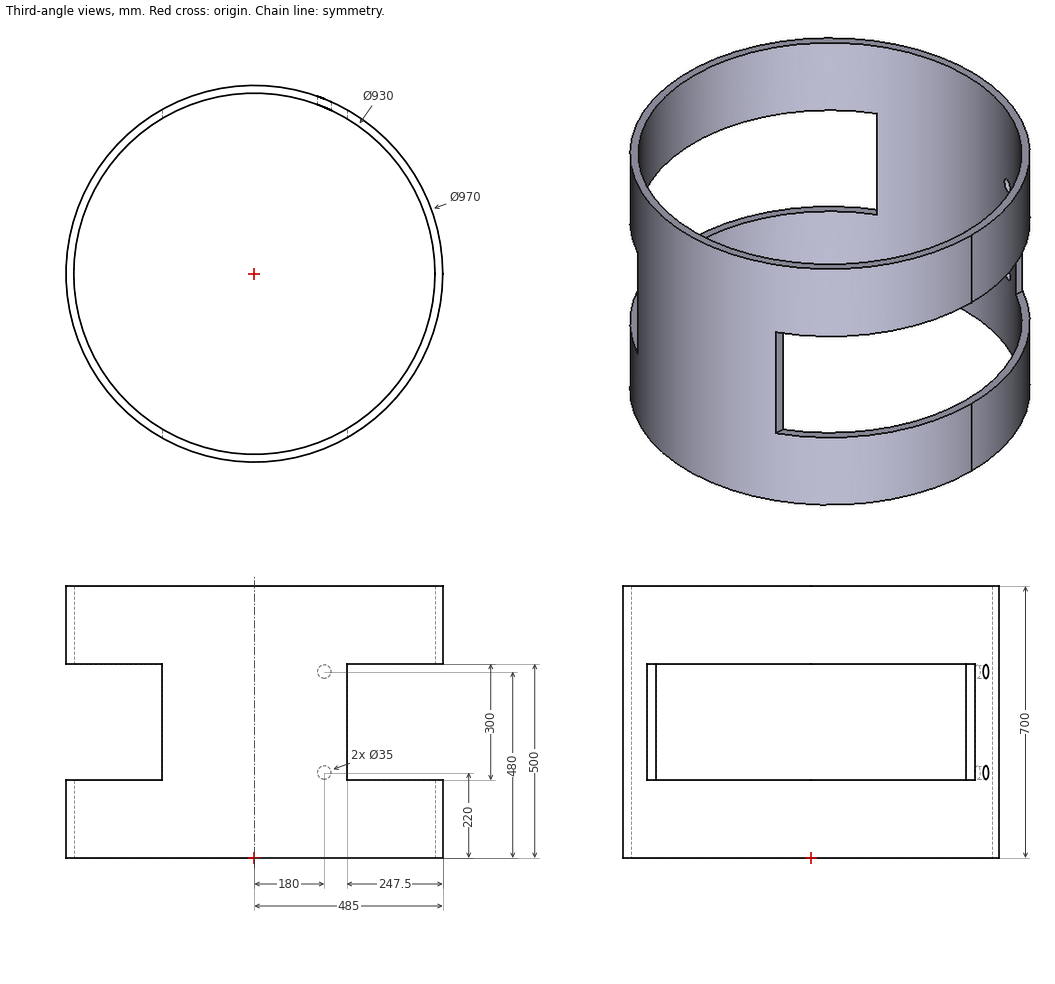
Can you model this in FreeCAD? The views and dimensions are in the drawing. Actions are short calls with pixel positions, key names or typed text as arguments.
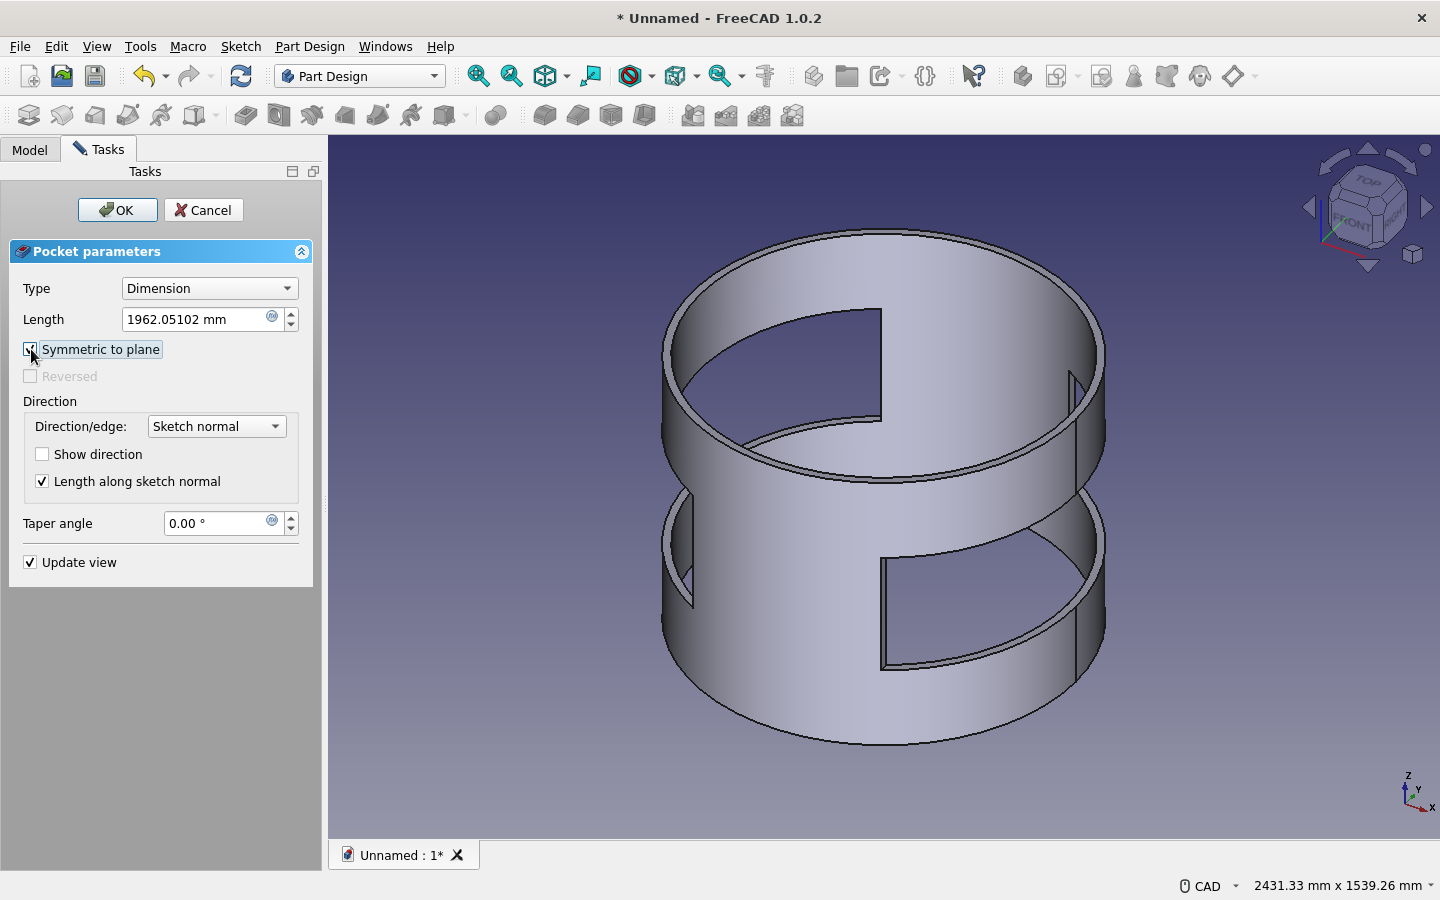
click(118, 210)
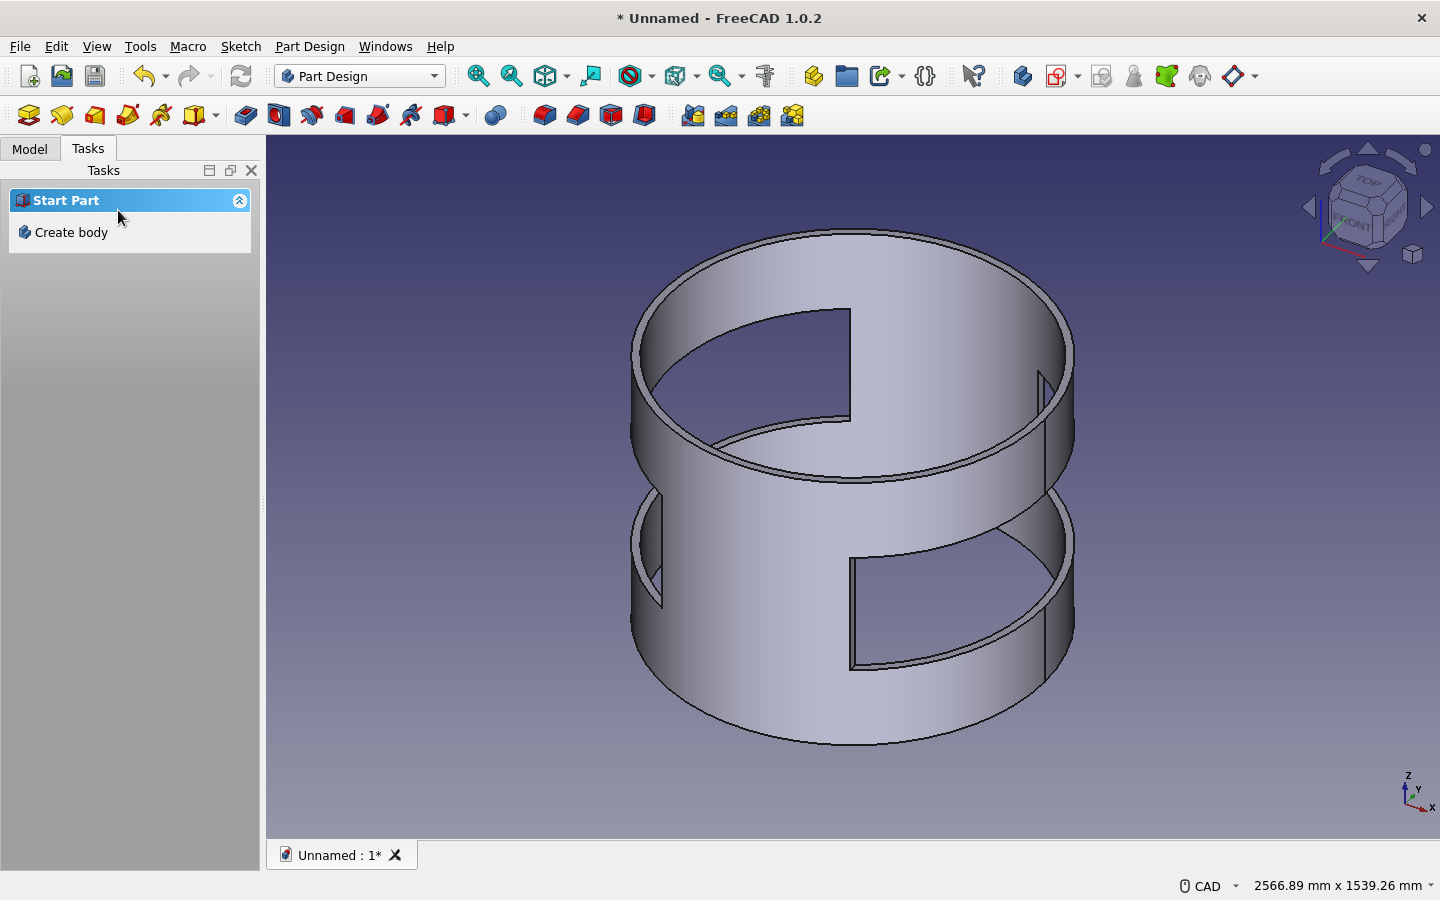
click(1056, 76)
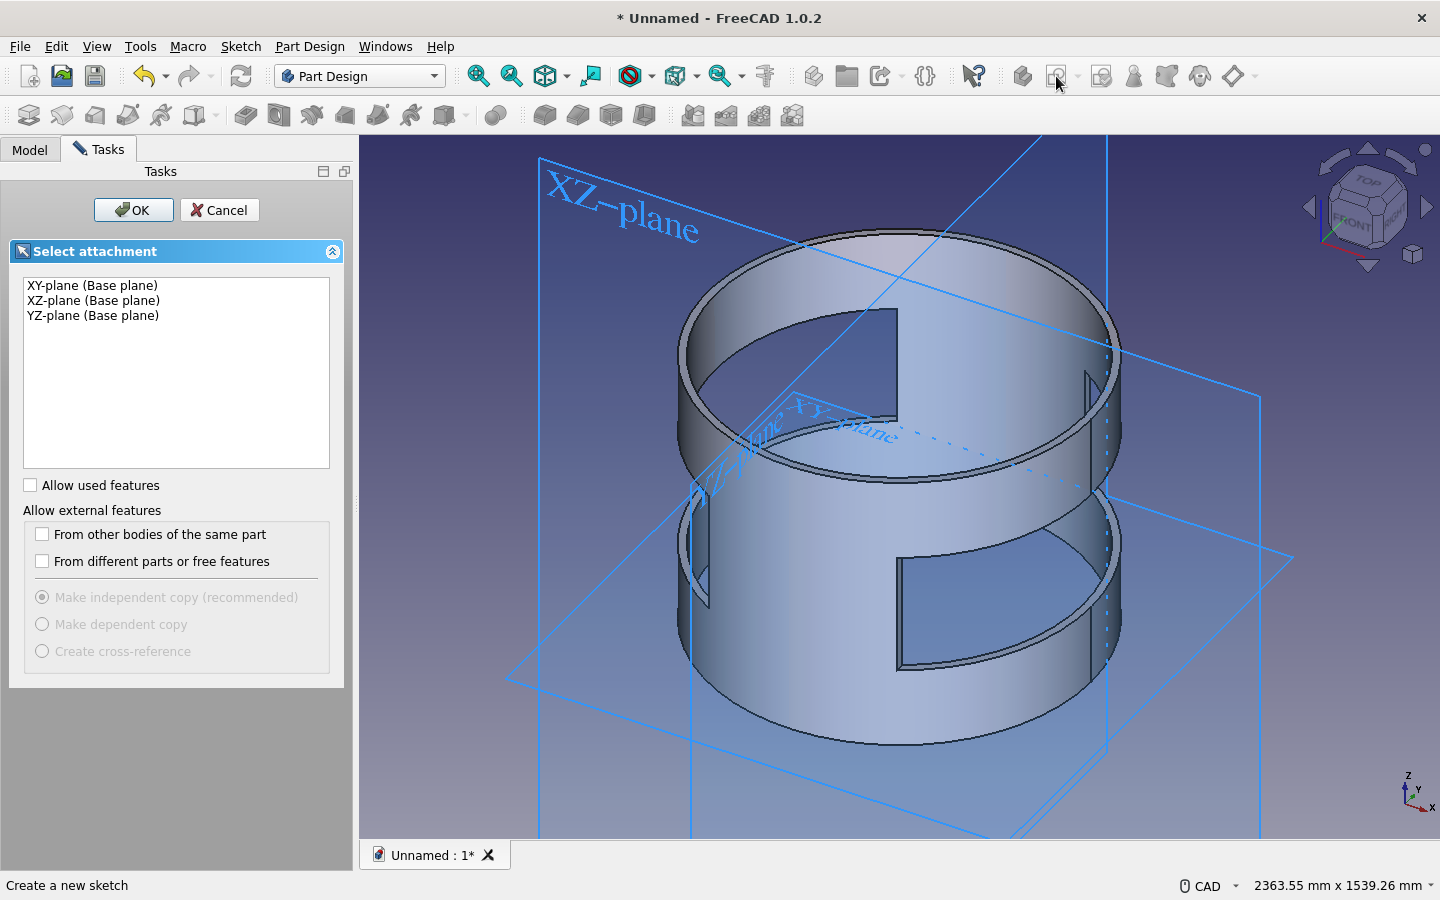
click(84, 300)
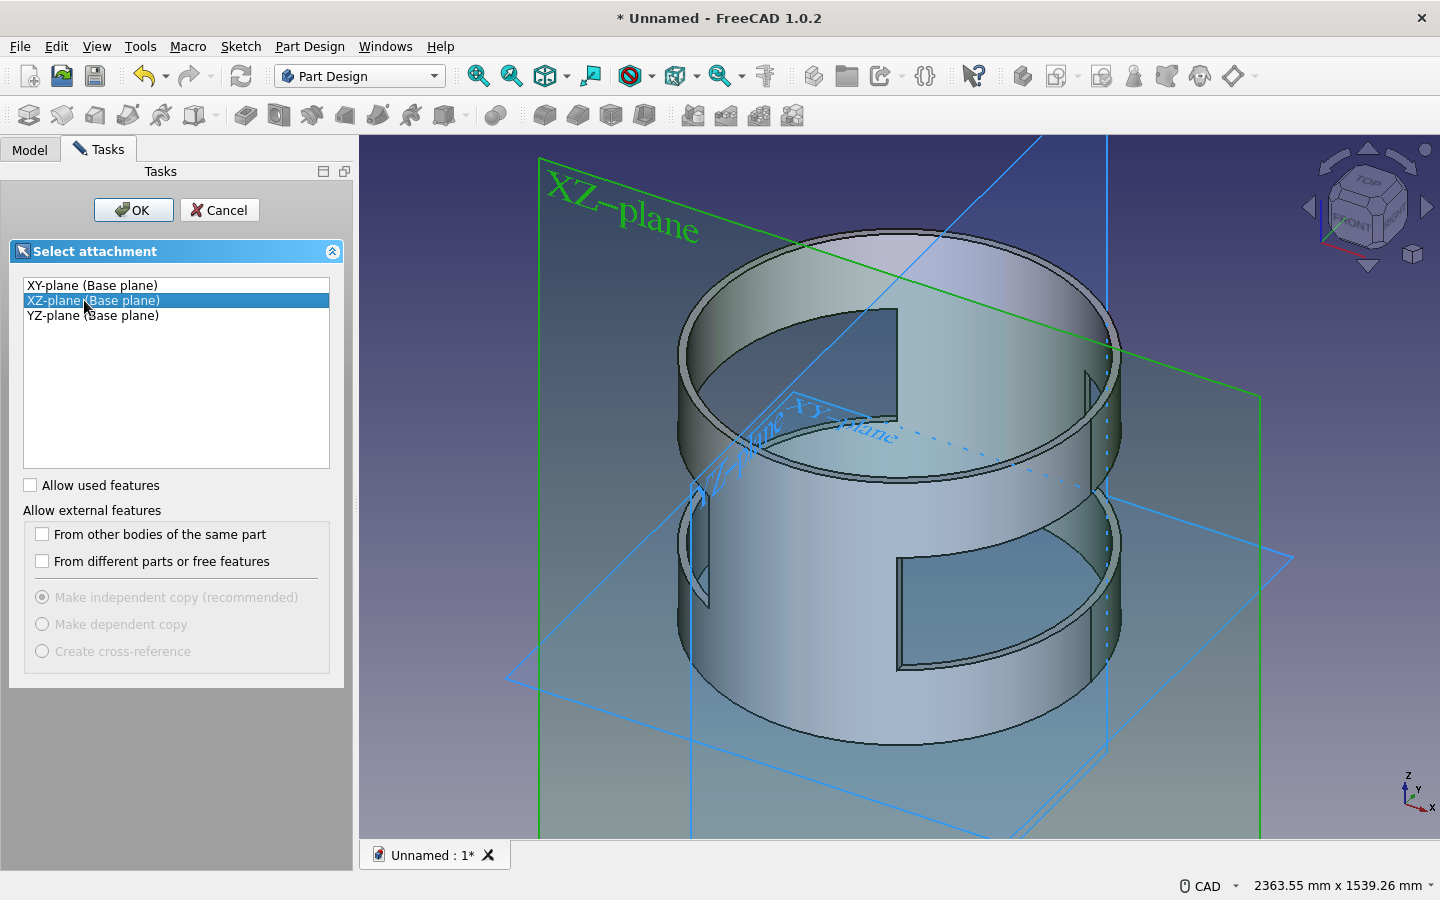
click(134, 210)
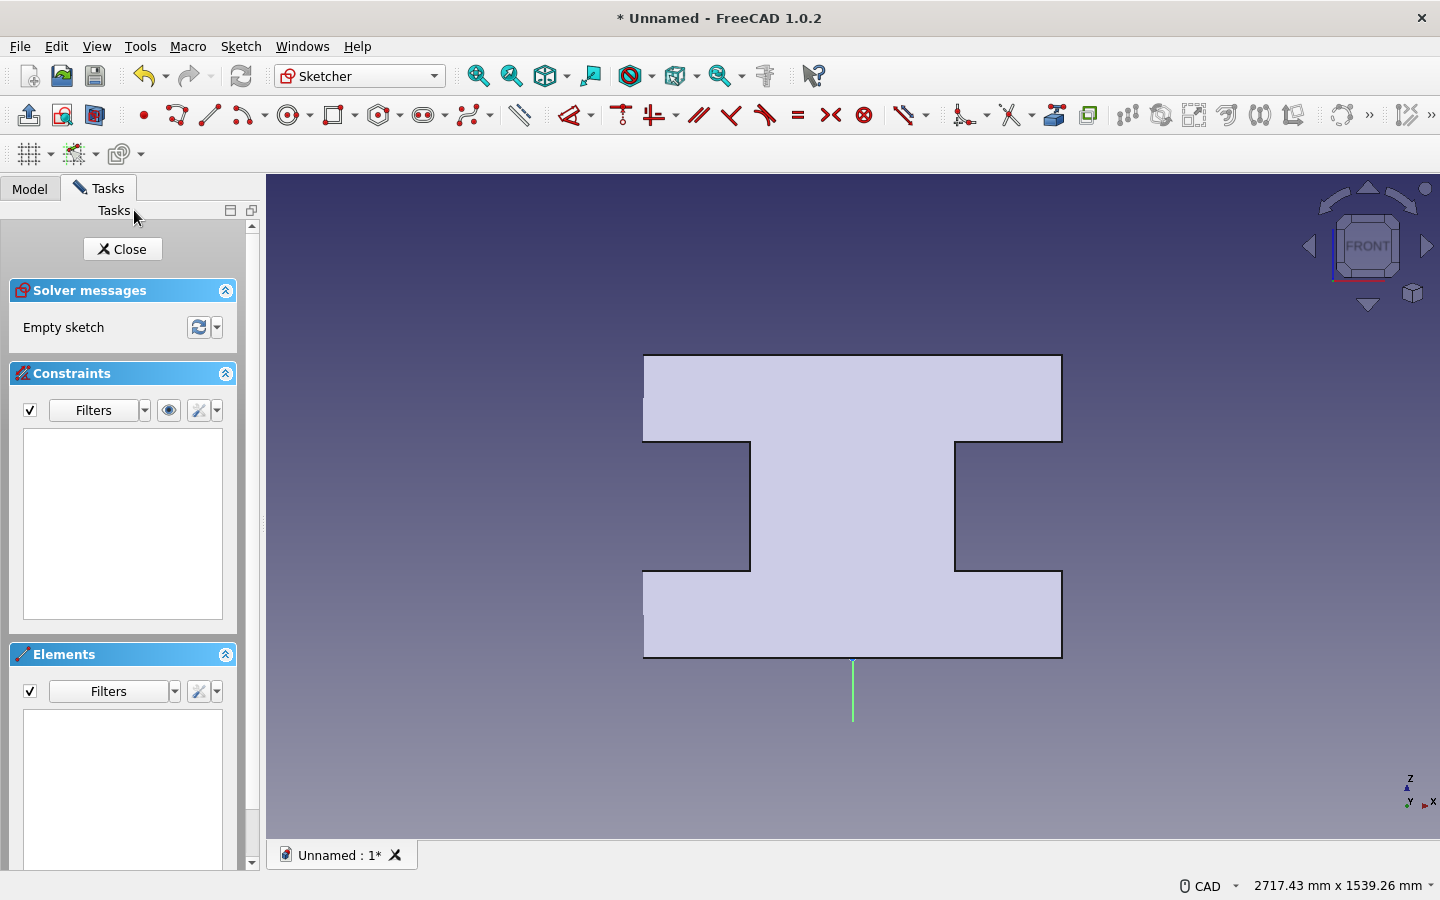
key(q)
key(s)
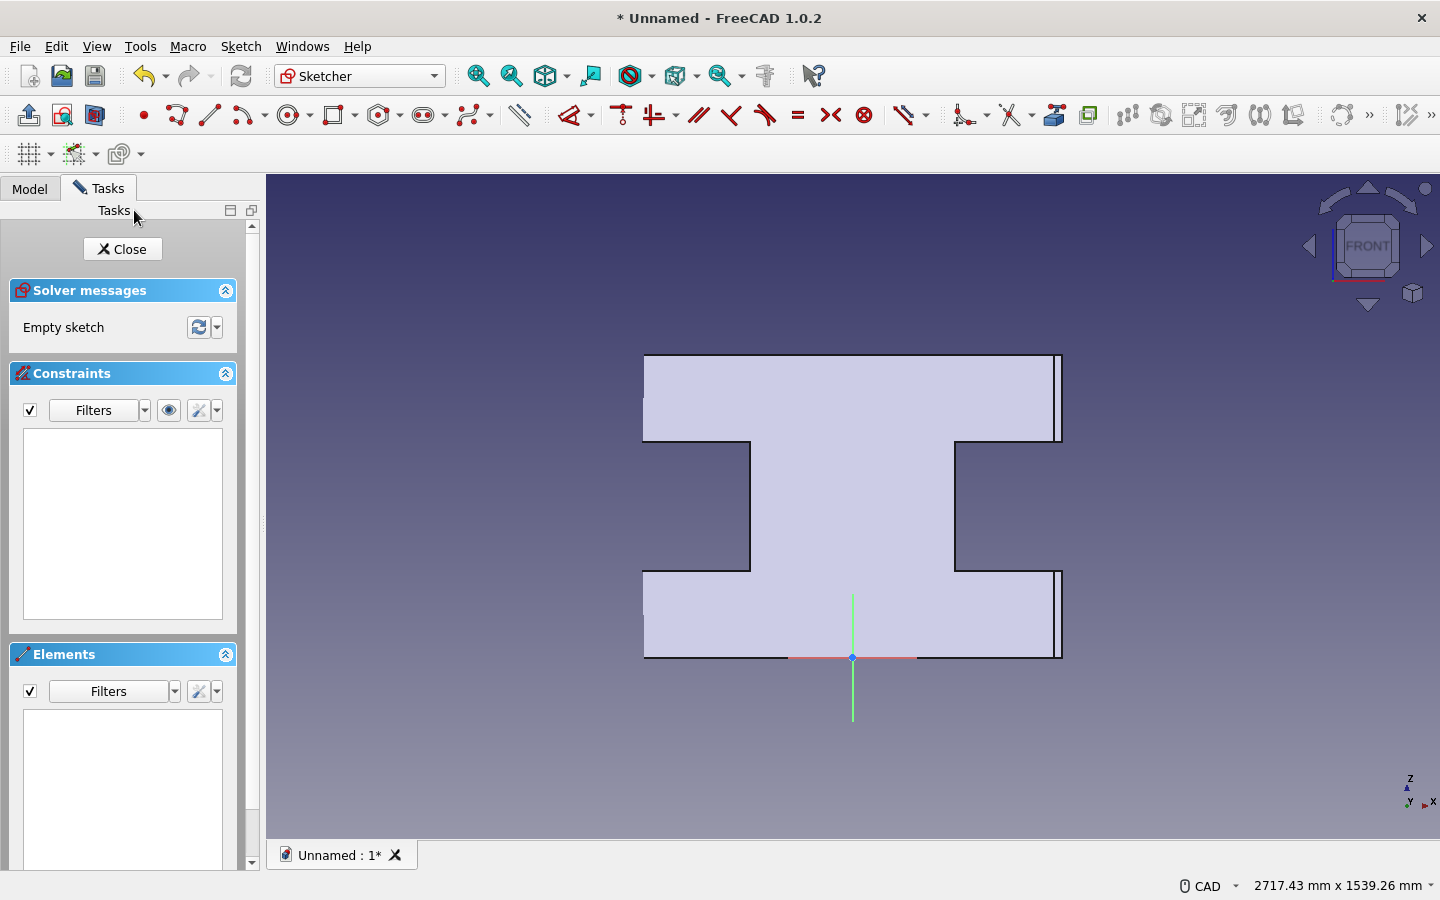
scroll(1031, 603, up, 3)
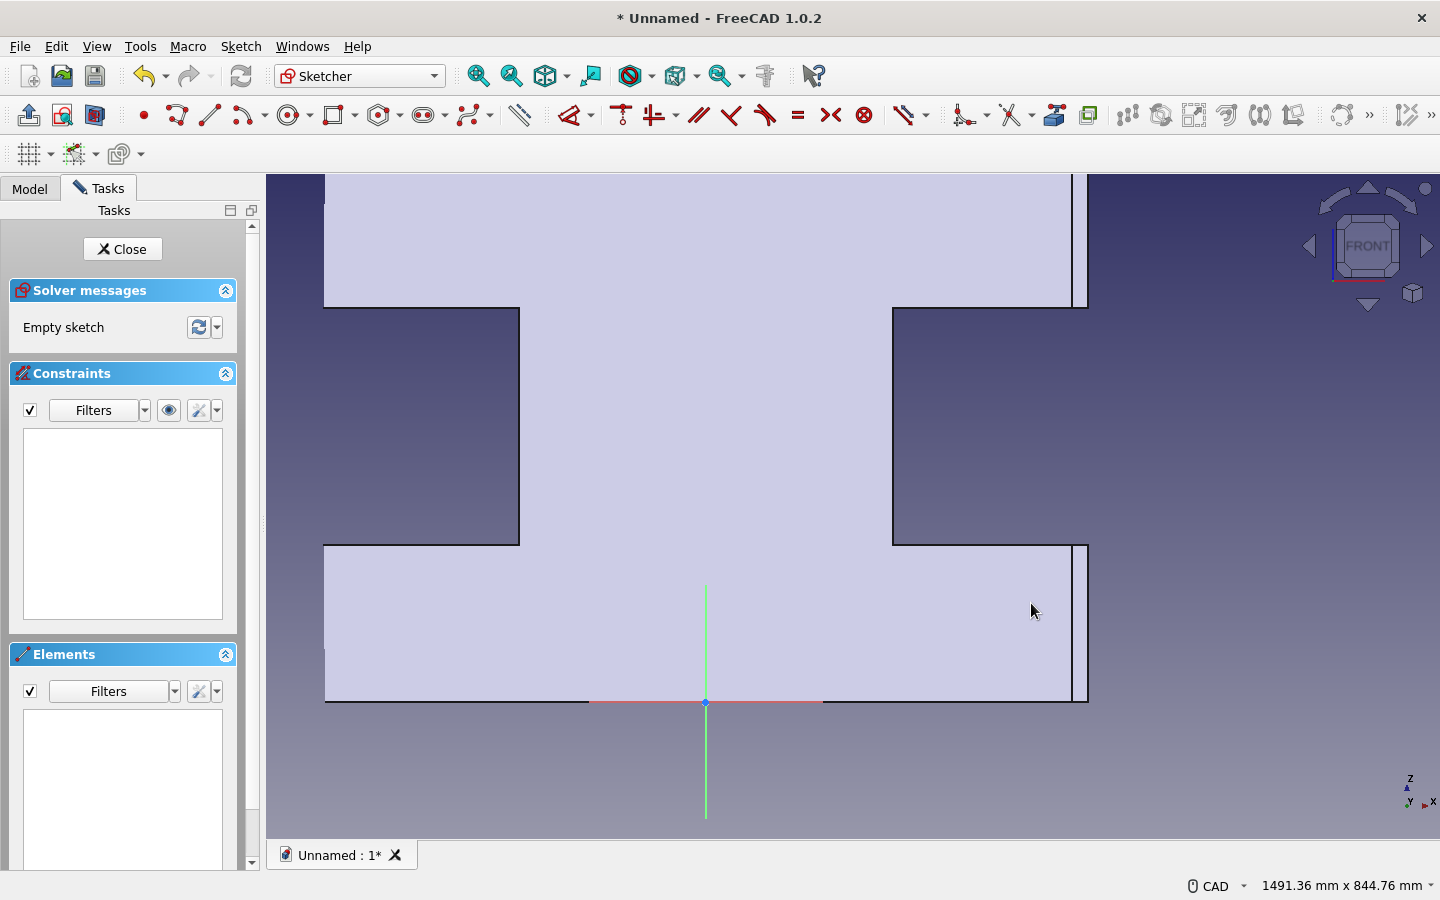
click(288, 116)